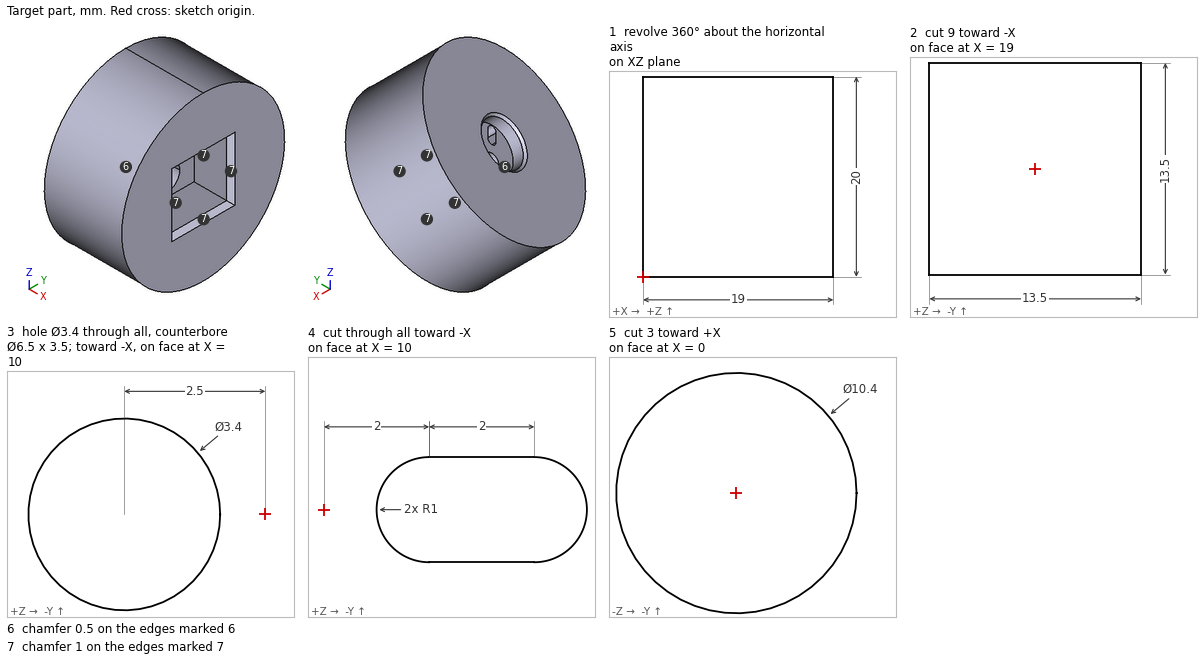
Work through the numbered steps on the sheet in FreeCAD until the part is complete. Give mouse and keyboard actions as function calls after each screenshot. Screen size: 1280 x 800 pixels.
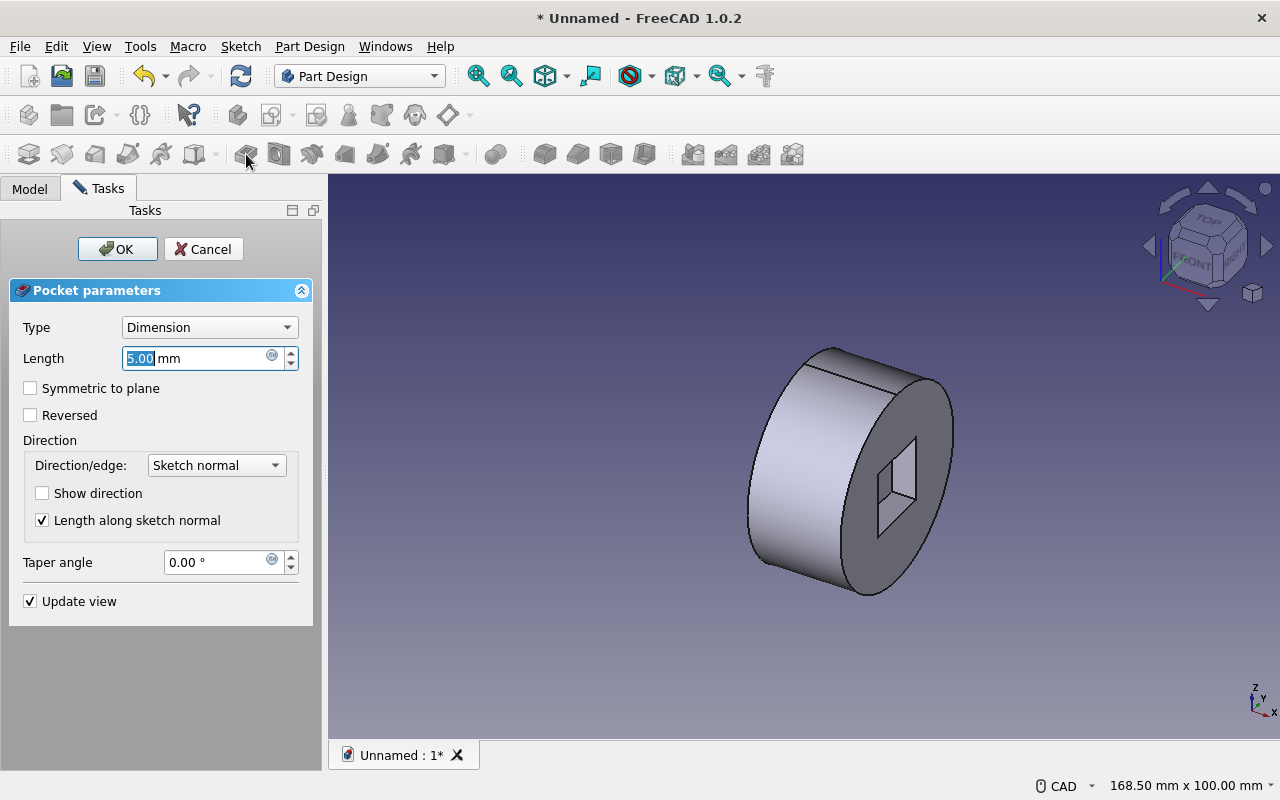
text(9)
key(Tab)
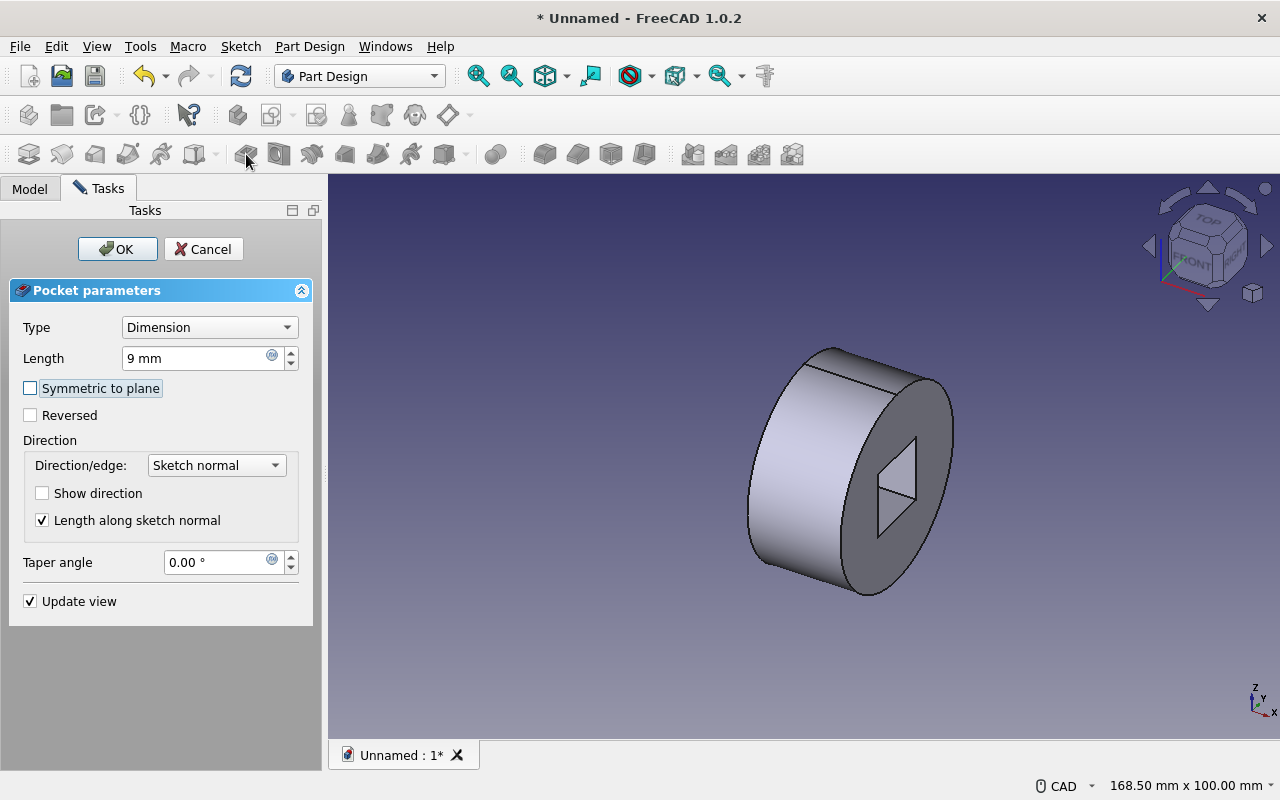
click(118, 249)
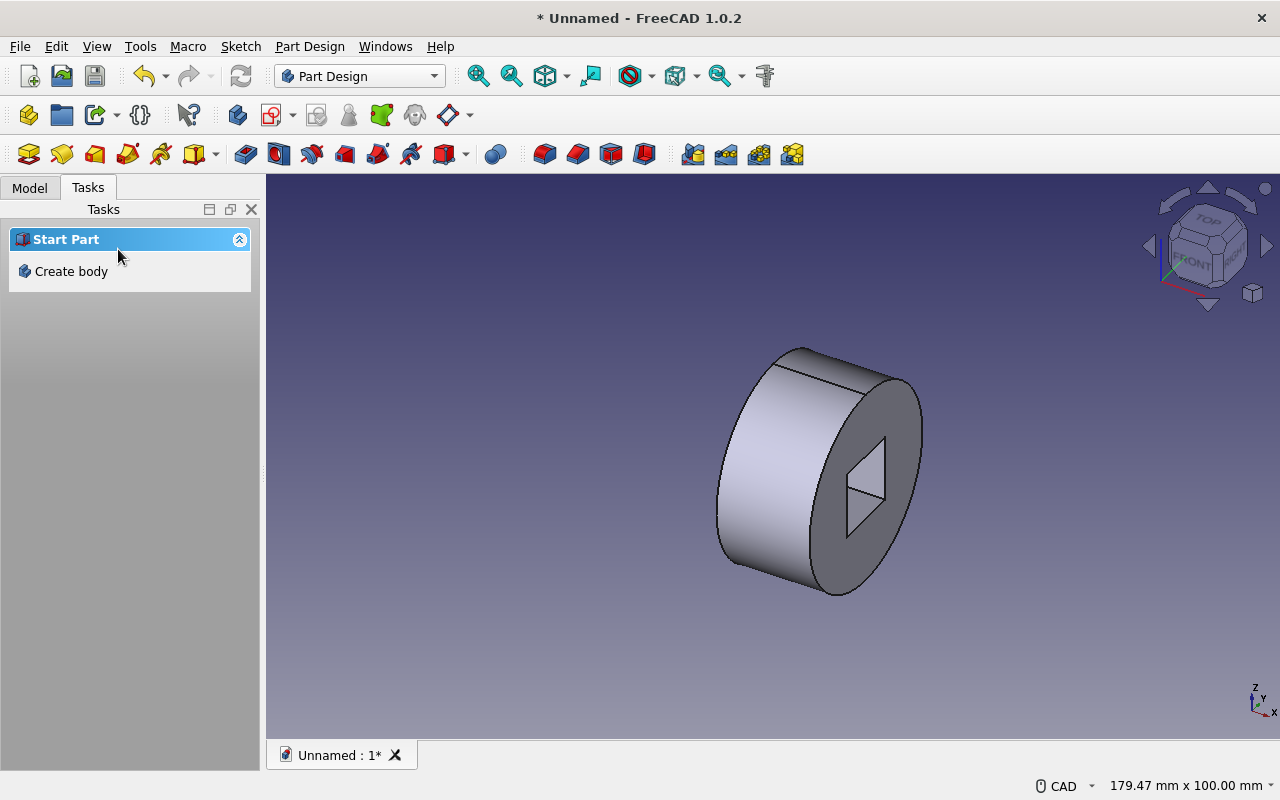
key(0)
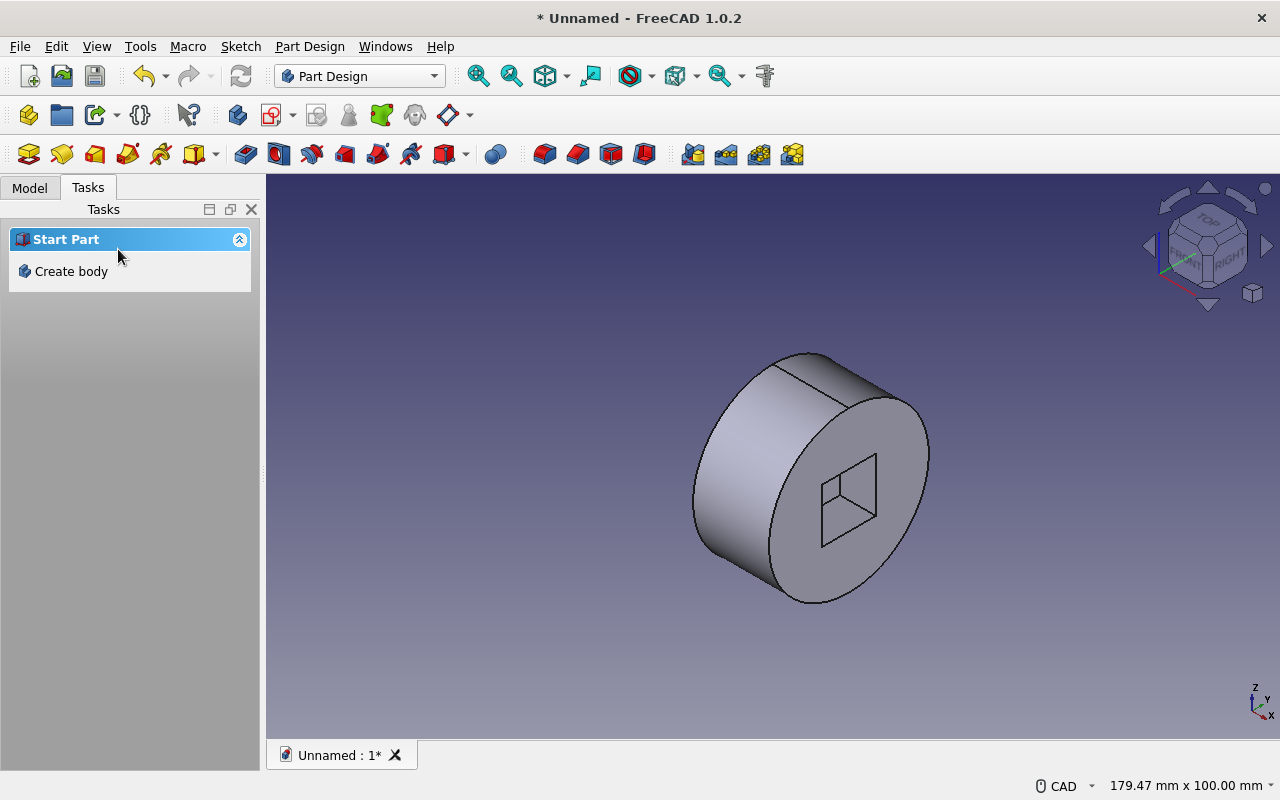
key(3)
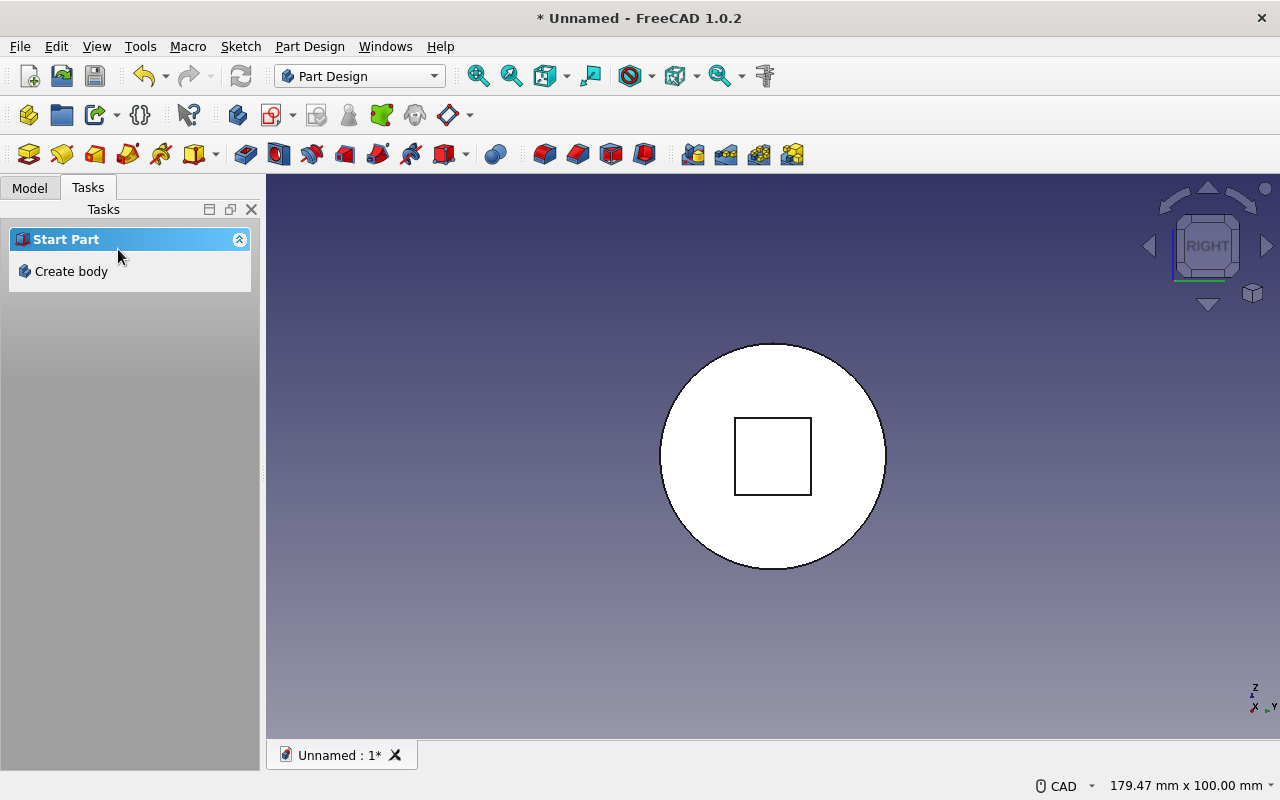
click(479, 76)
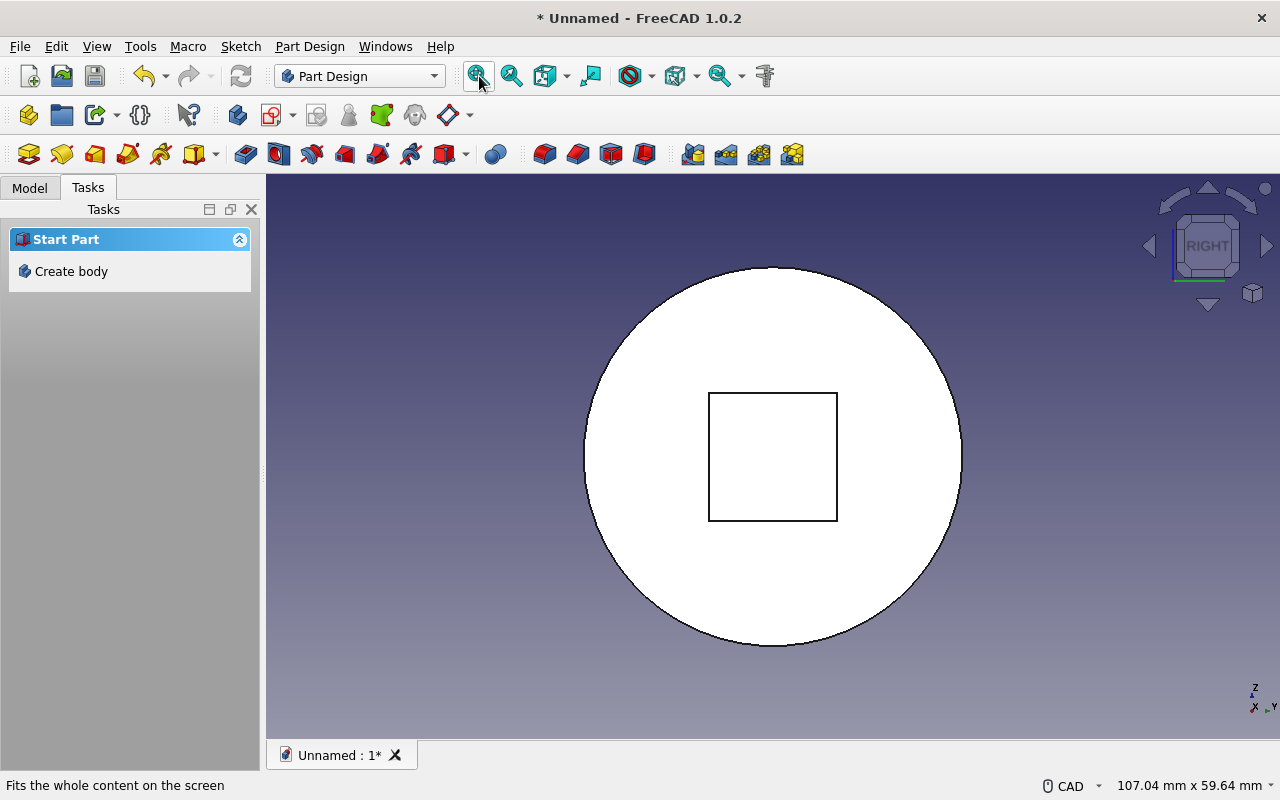
click(773, 456)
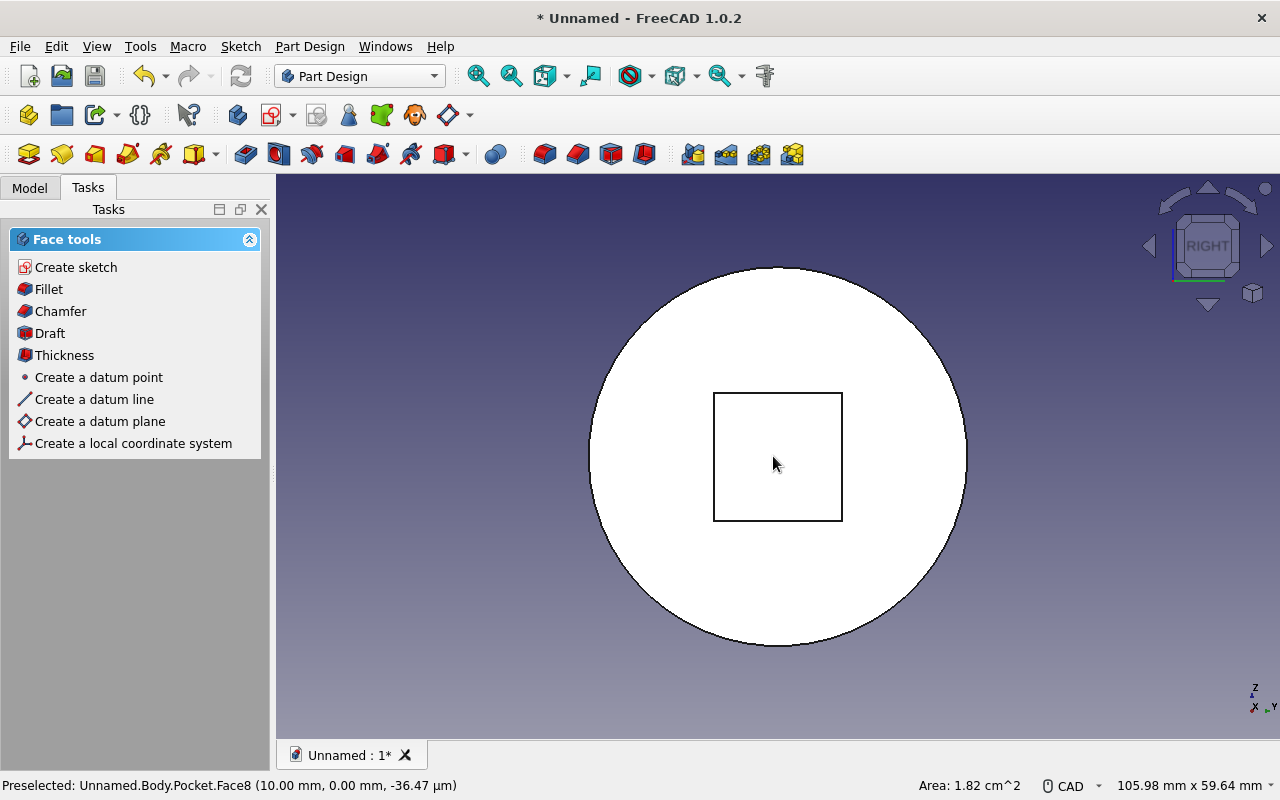
click(270, 116)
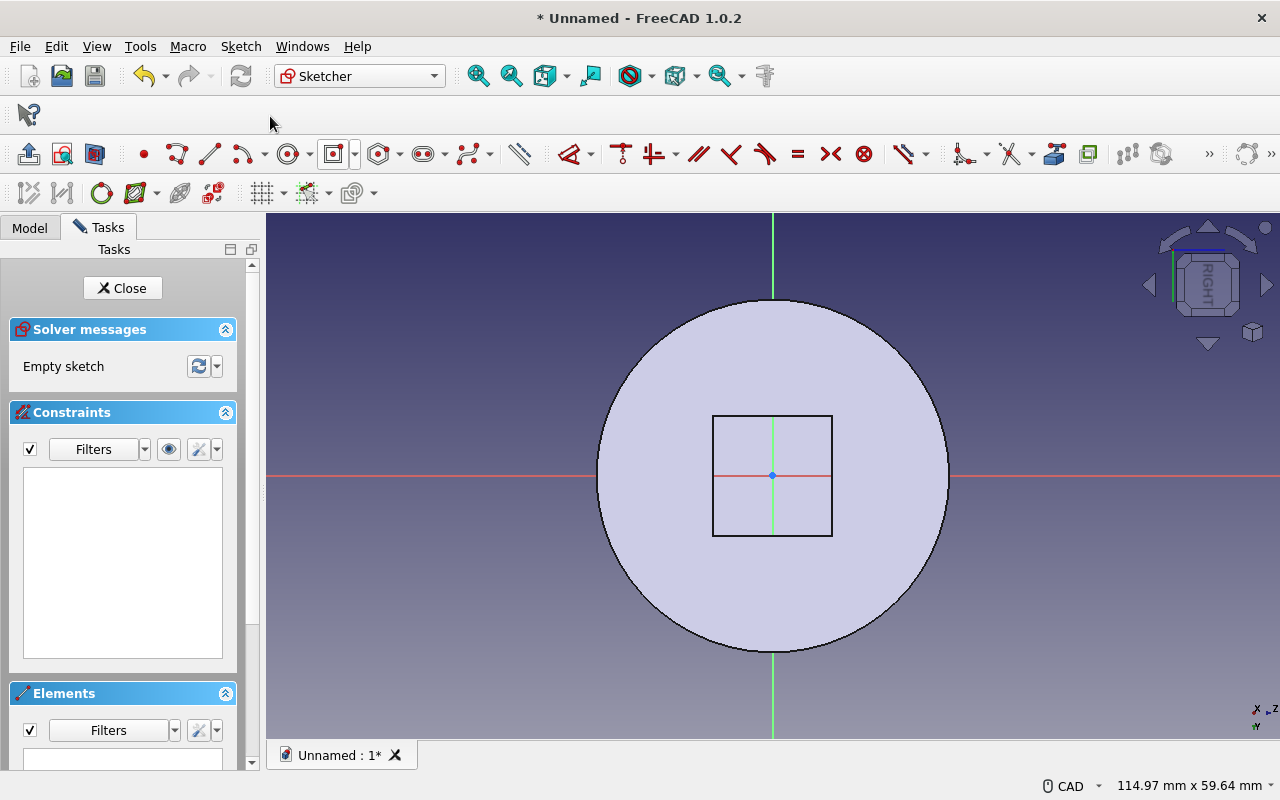
scroll(759, 476, up, 12)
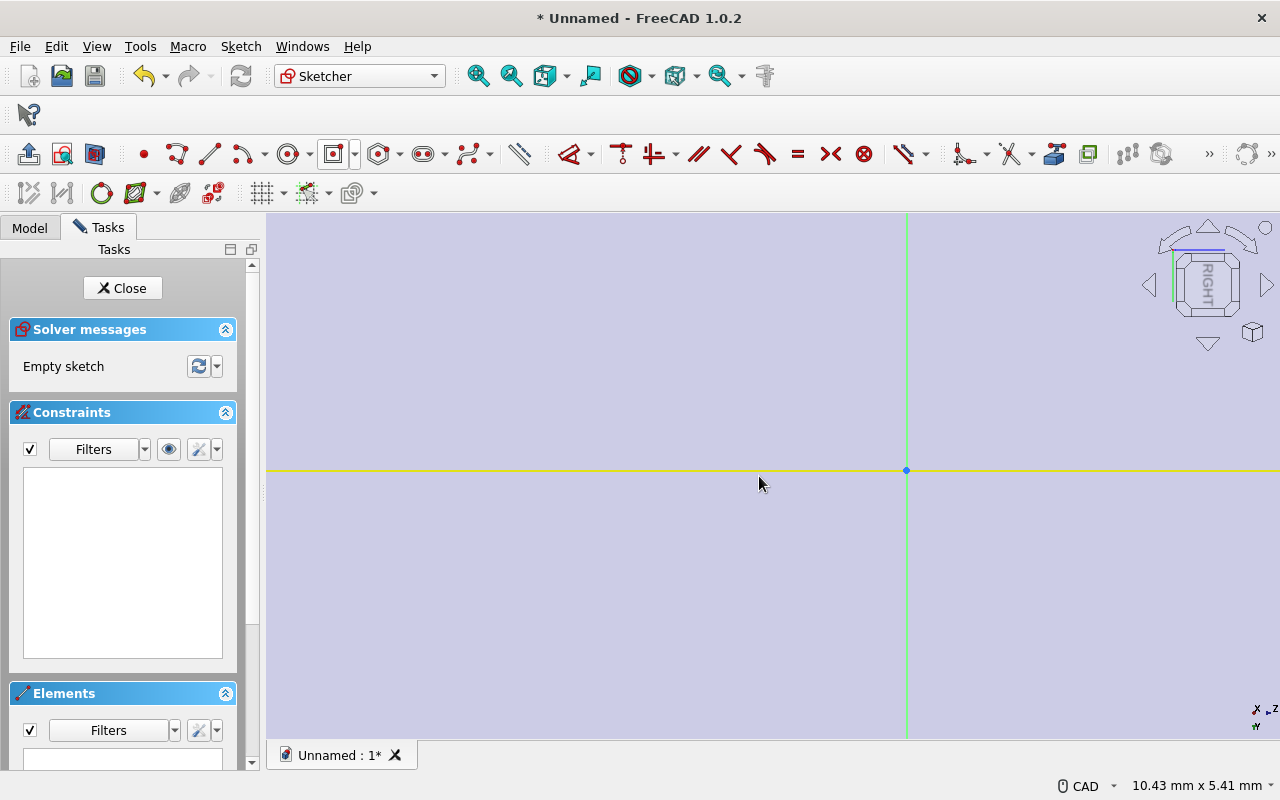
click(288, 154)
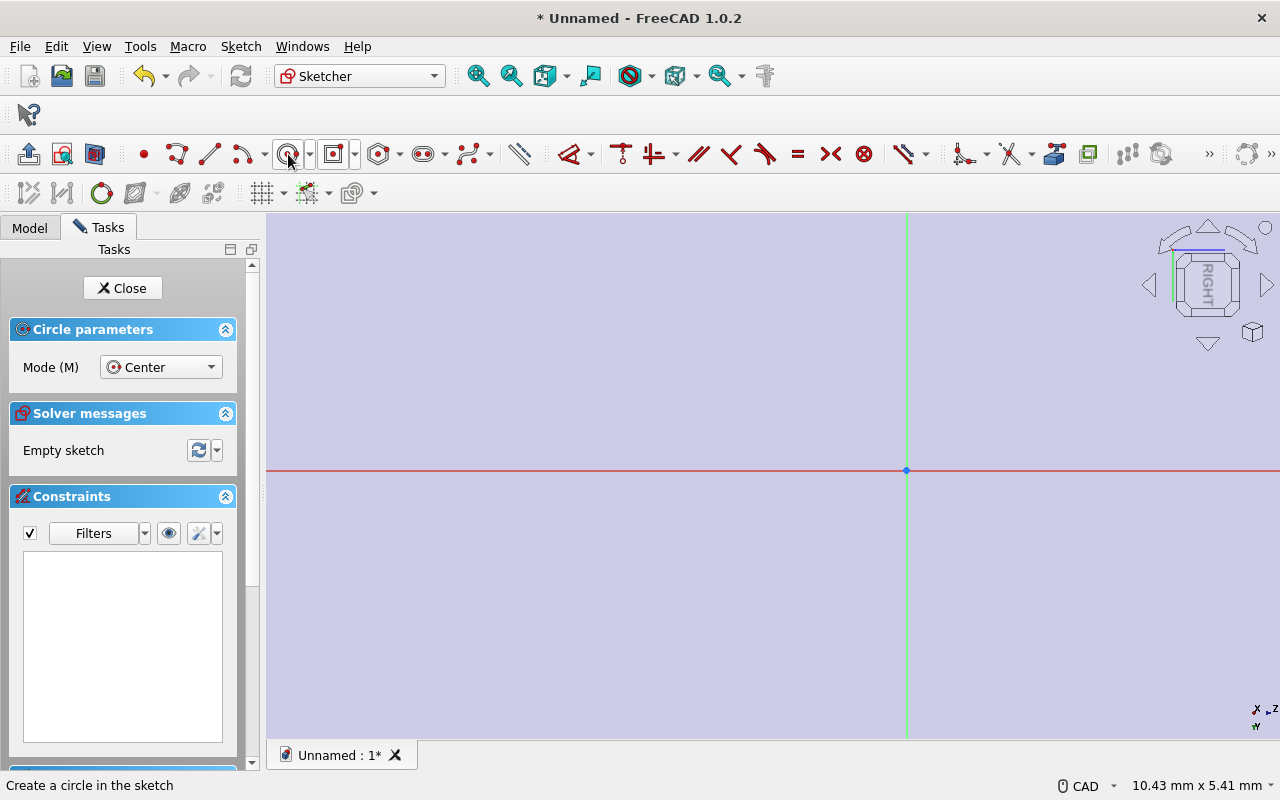
click(664, 471)
click(781, 354)
key(Escape)